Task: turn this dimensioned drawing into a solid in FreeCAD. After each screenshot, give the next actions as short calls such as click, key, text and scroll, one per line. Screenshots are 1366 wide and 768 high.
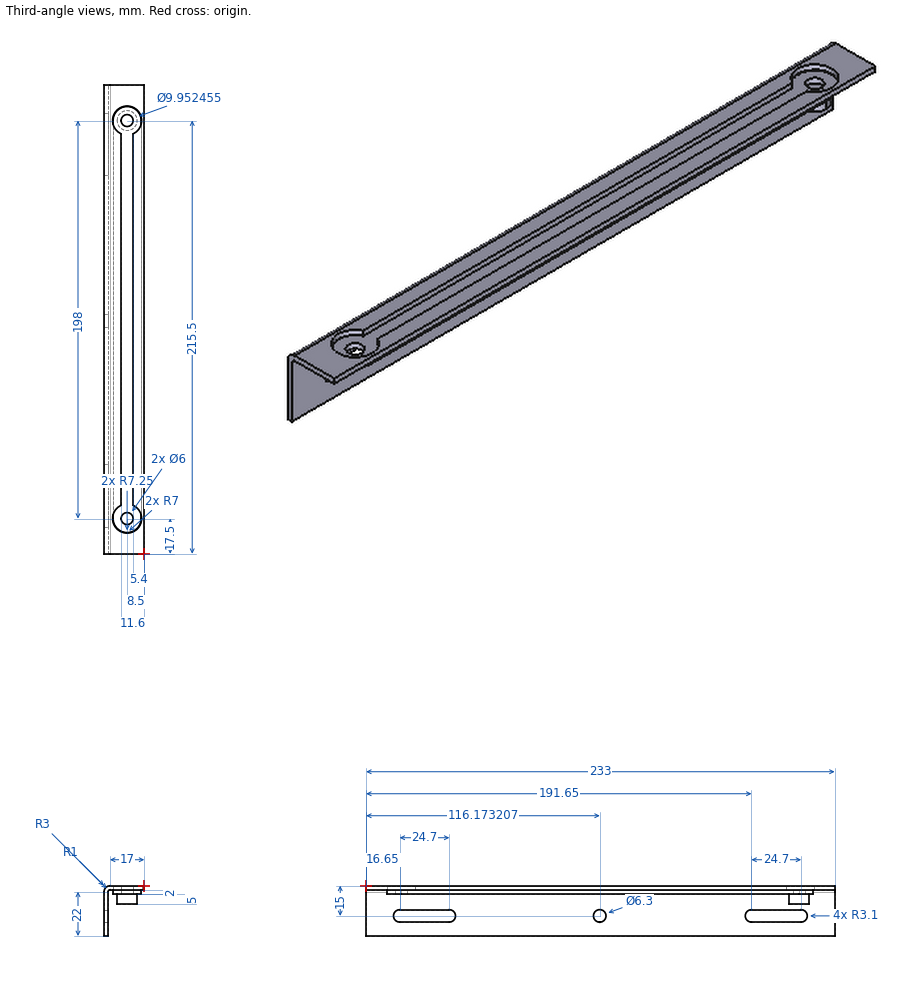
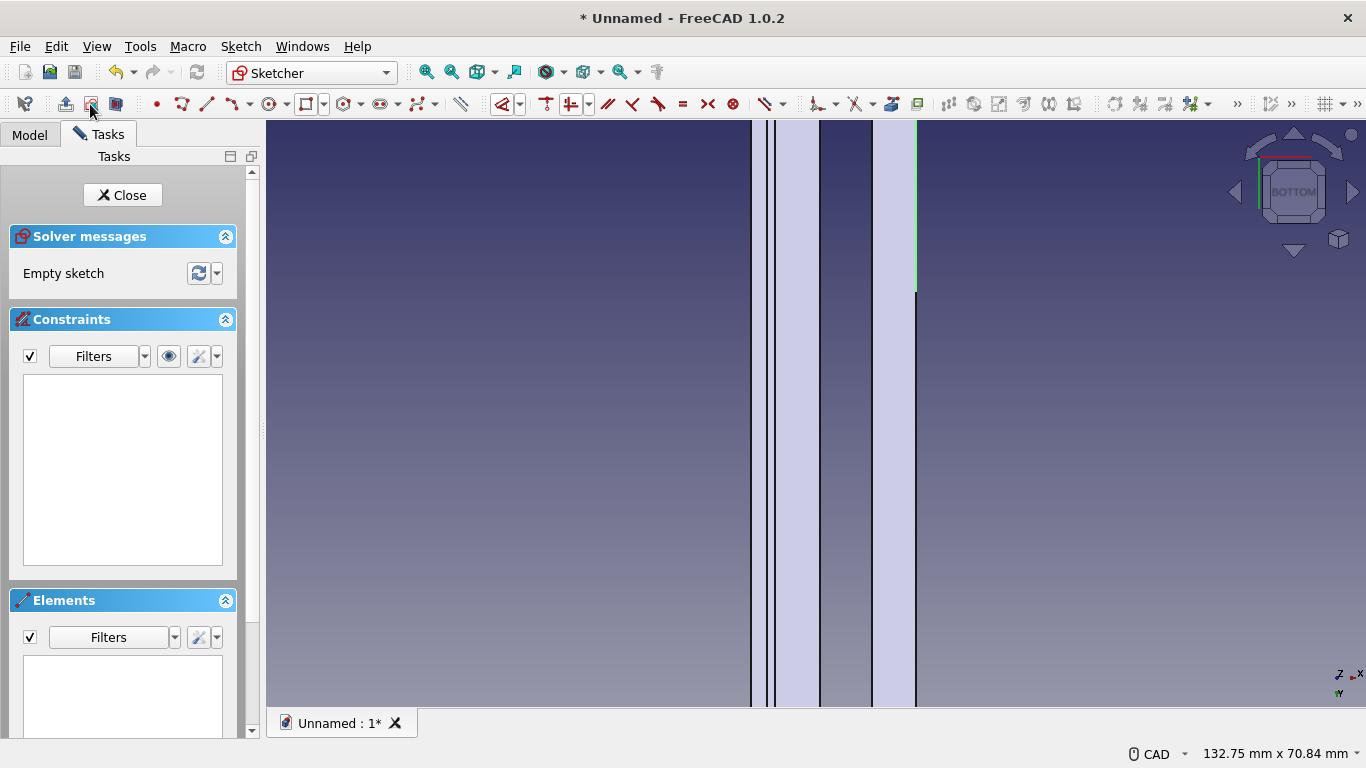
scroll(721, 522, down, 8)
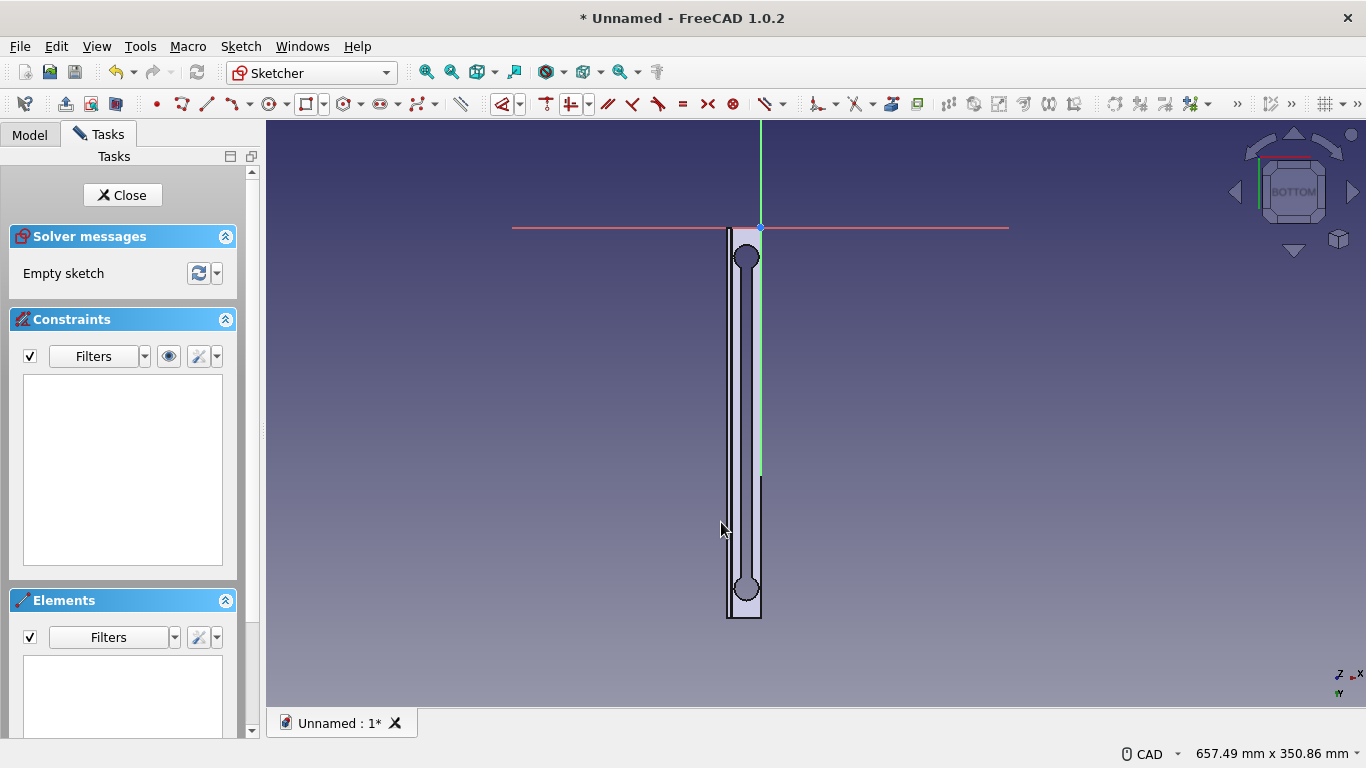
click(380, 104)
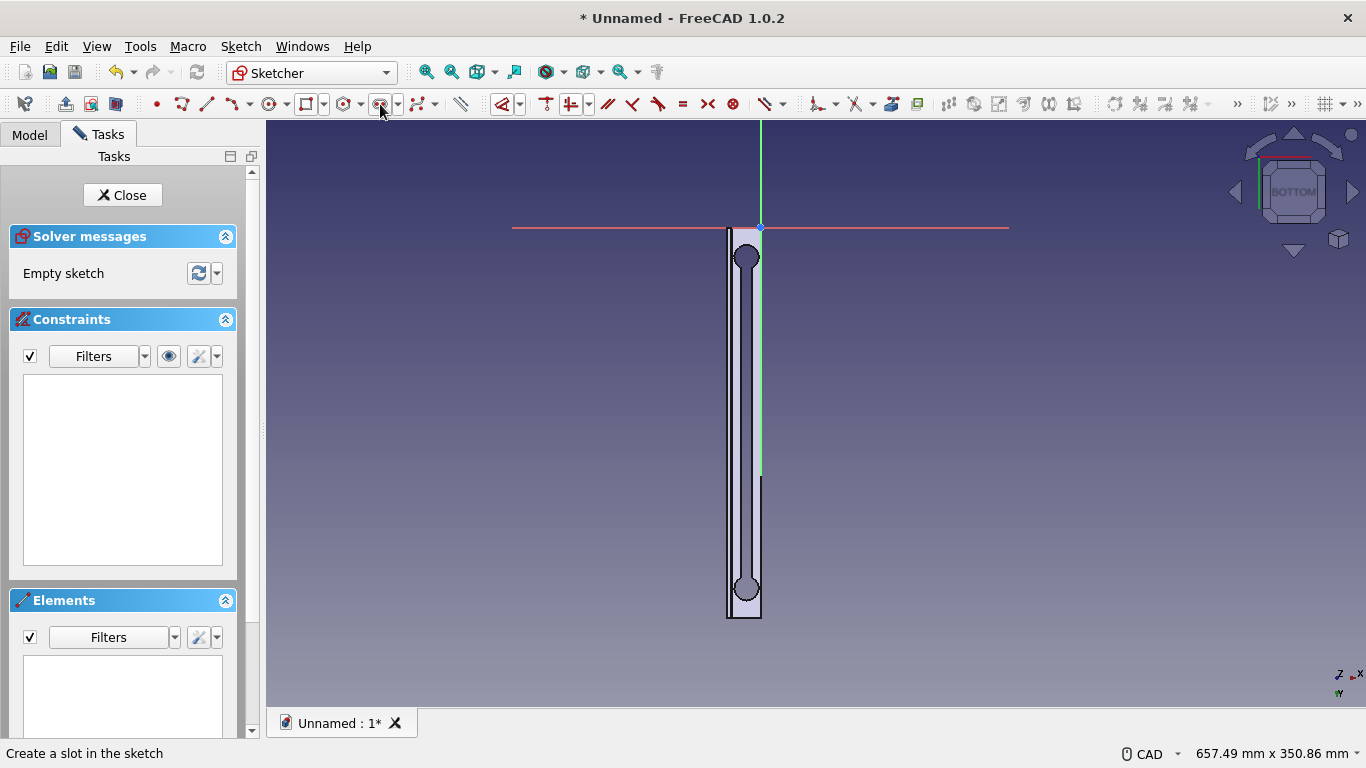
scroll(747, 588, up, 4)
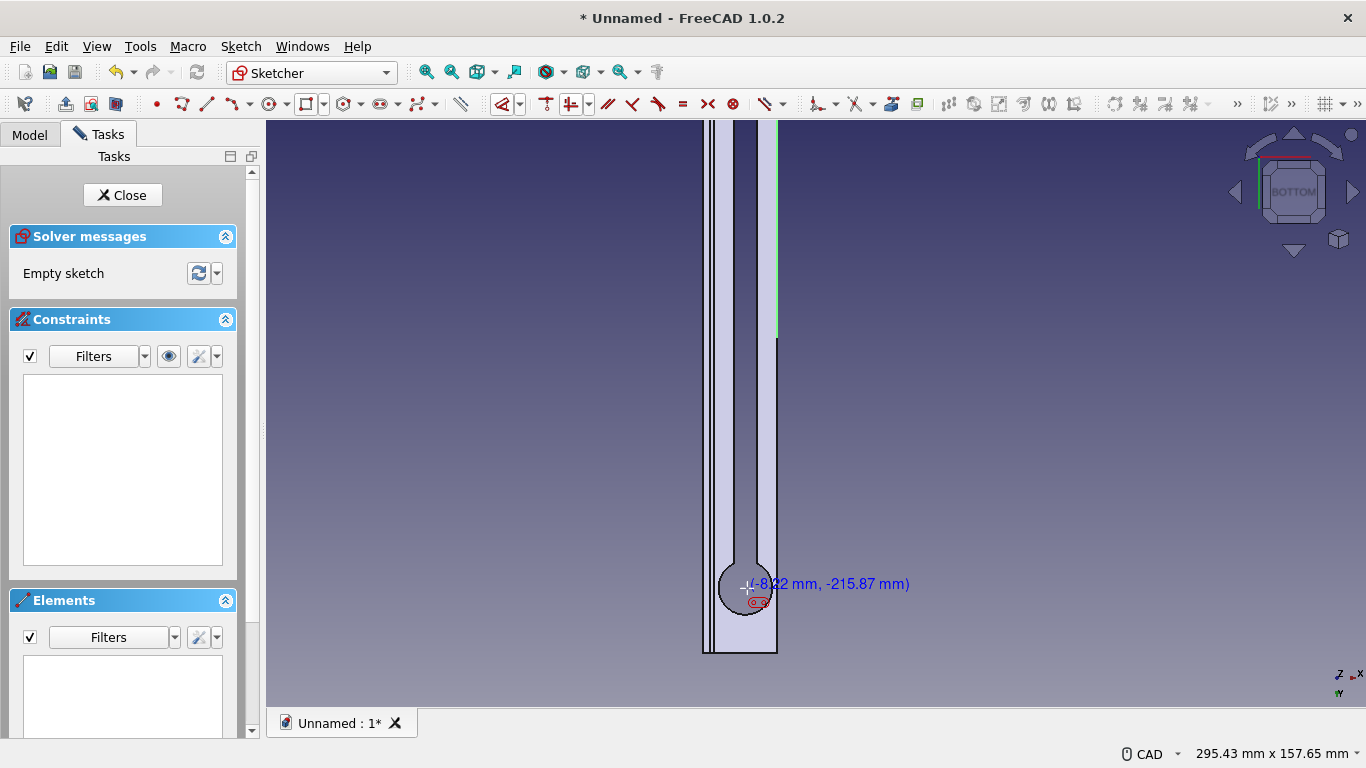
click(745, 588)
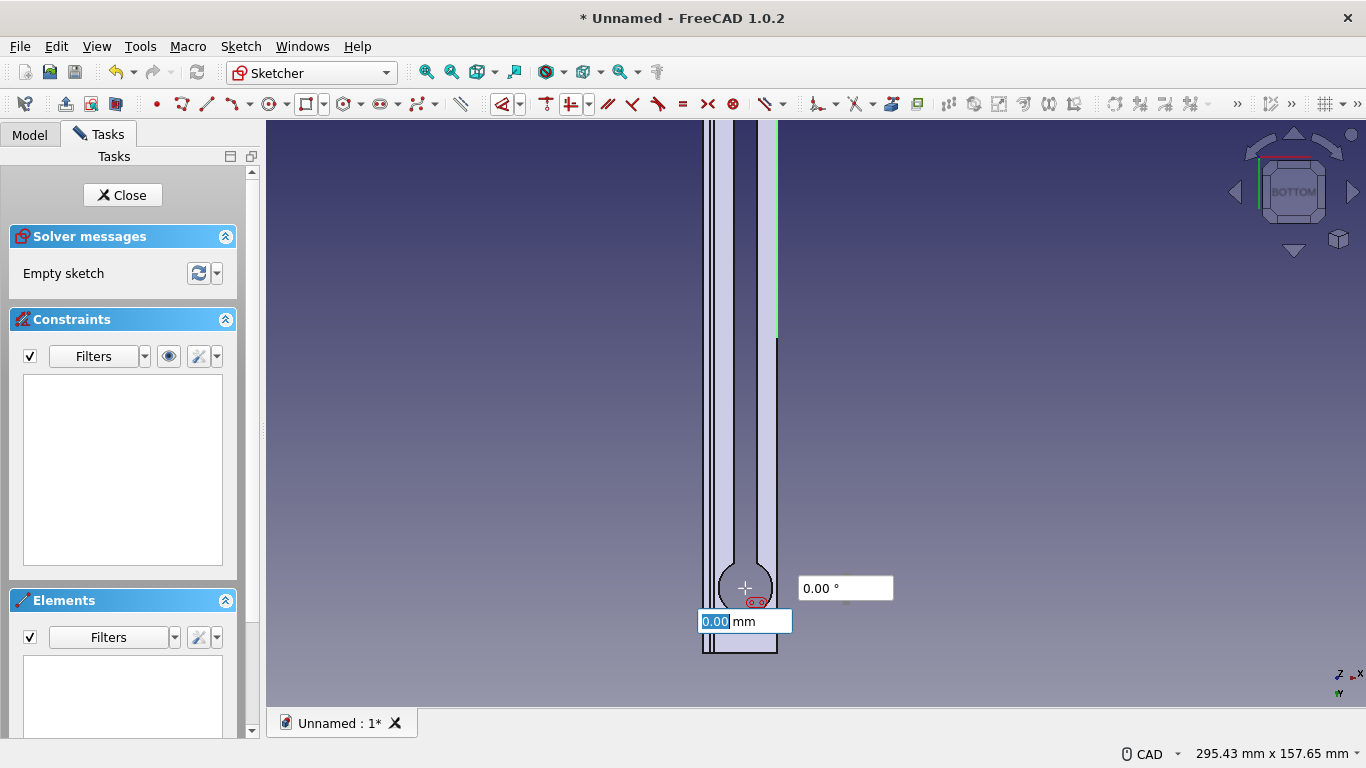
scroll(747, 588, down, 4)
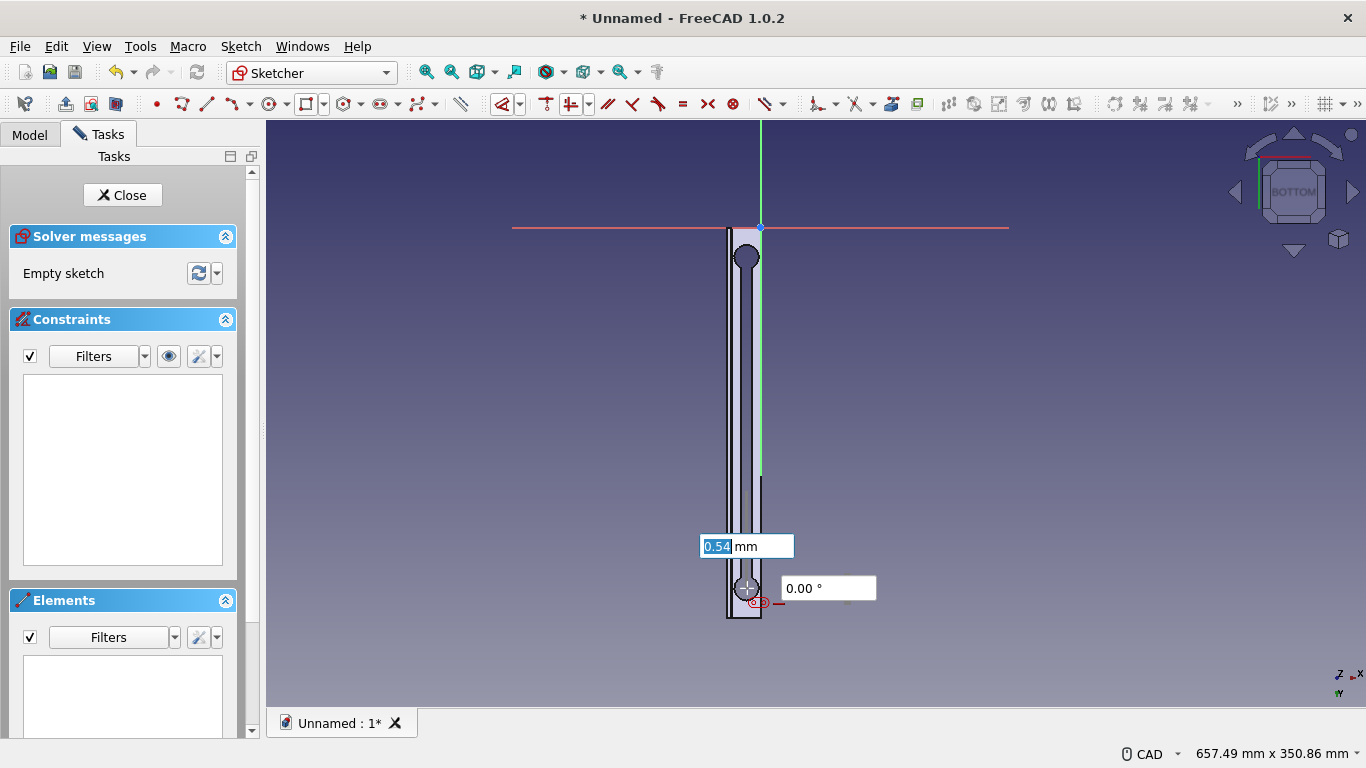
click(746, 257)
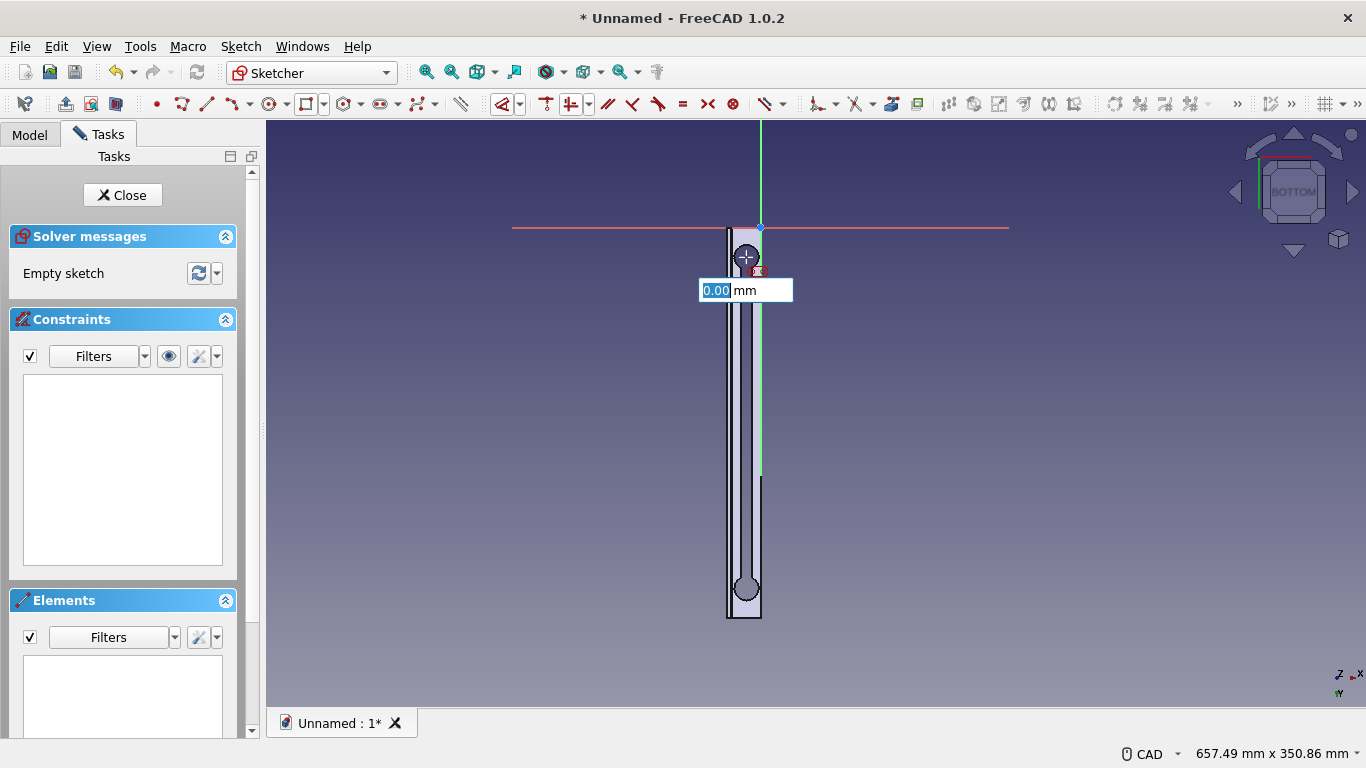
scroll(735, 423, up, 2)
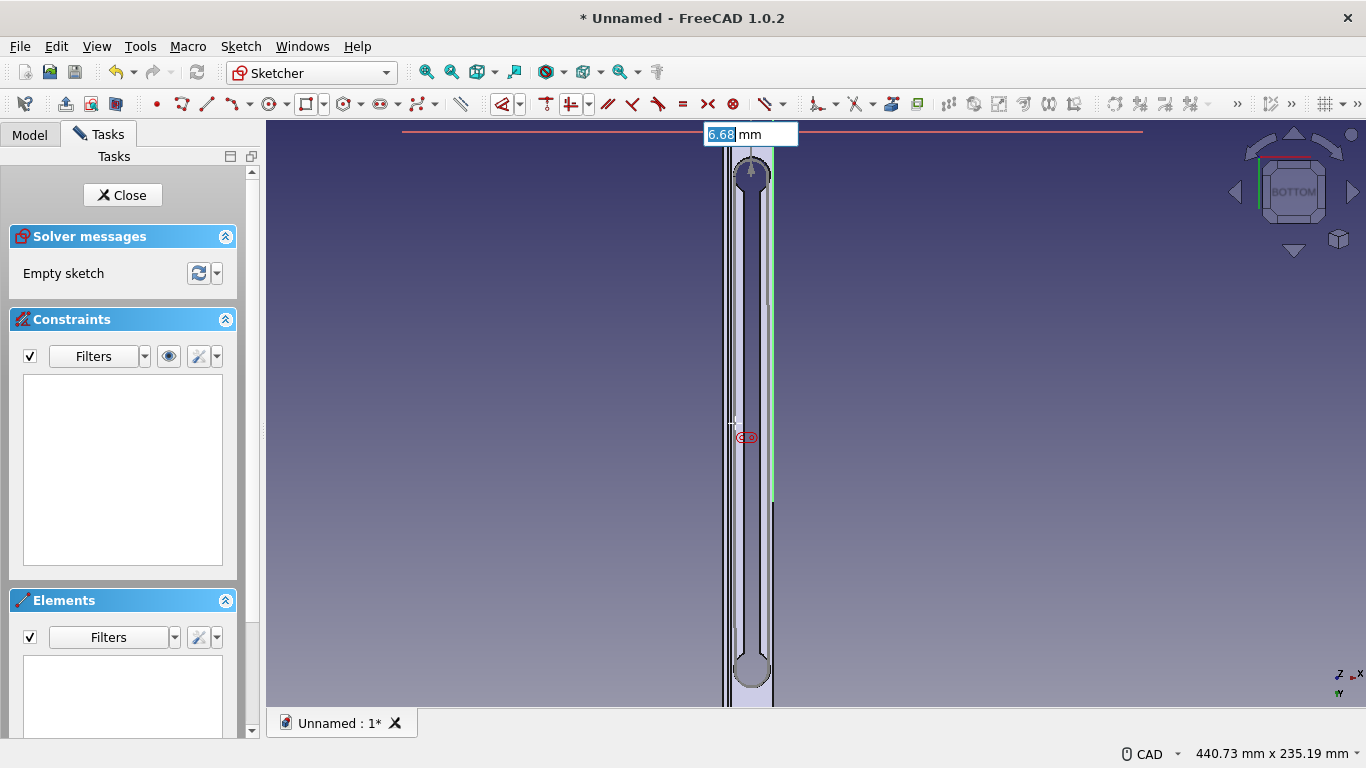
click(735, 422)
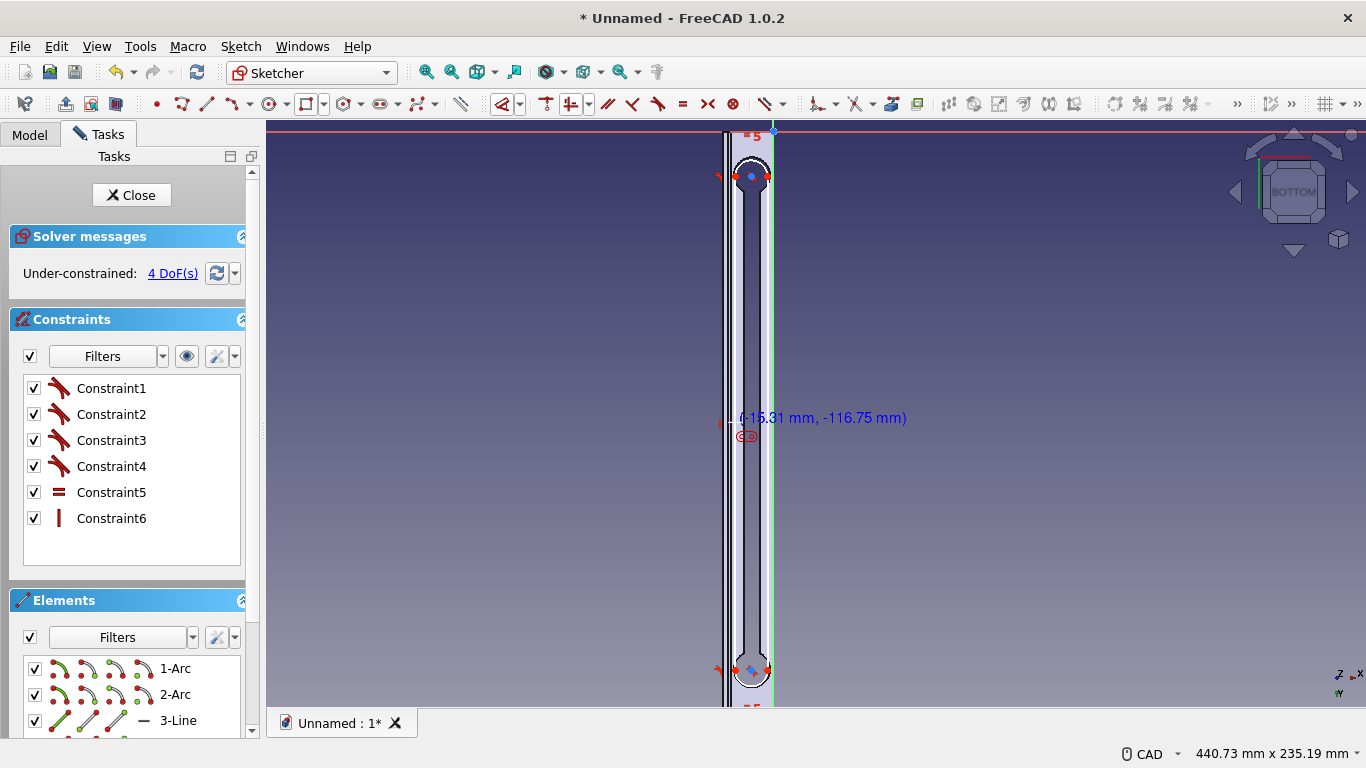
click(268, 104)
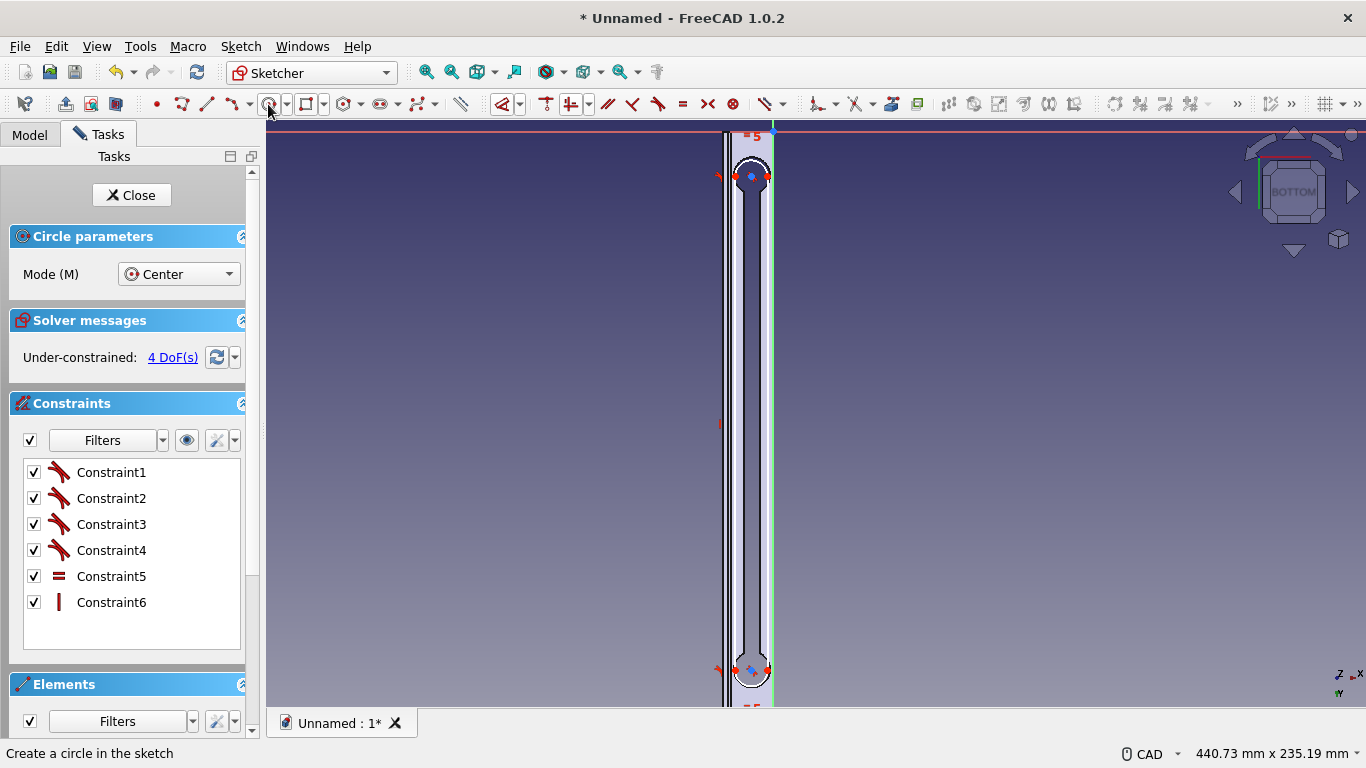
scroll(752, 175, up, 6)